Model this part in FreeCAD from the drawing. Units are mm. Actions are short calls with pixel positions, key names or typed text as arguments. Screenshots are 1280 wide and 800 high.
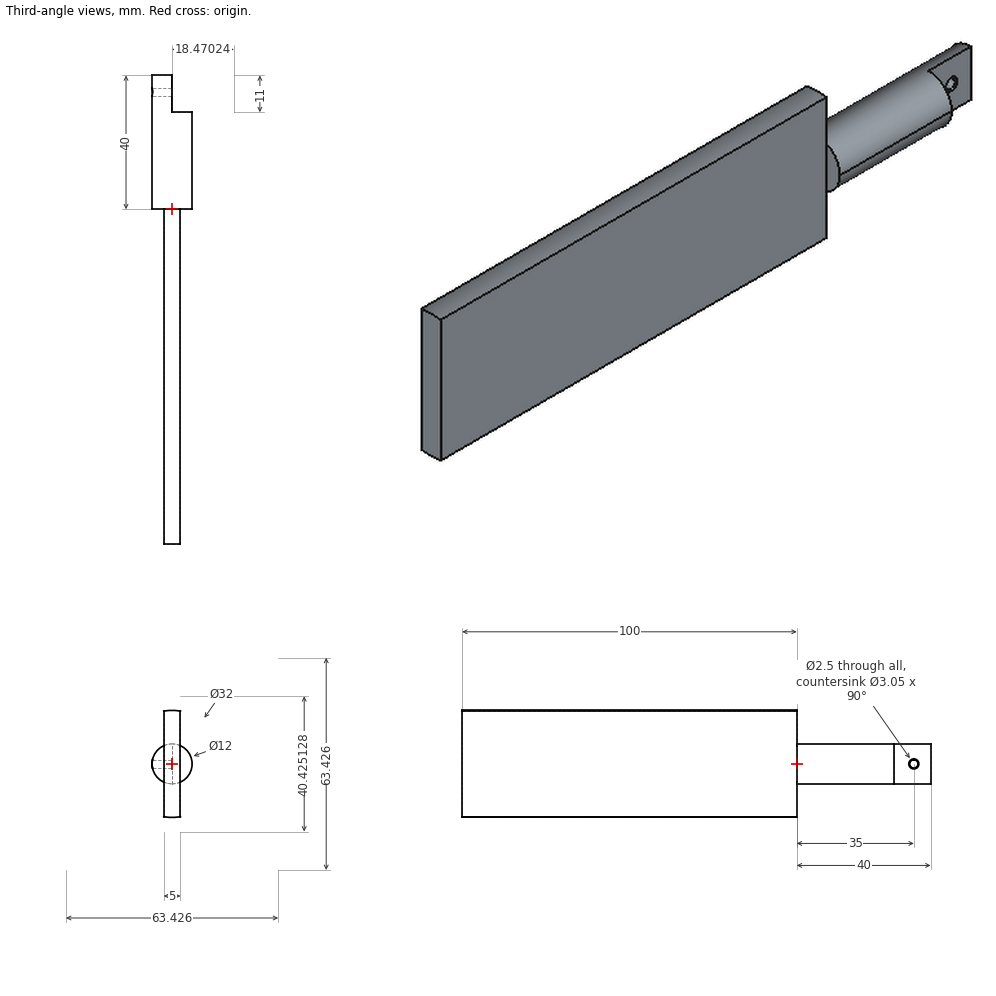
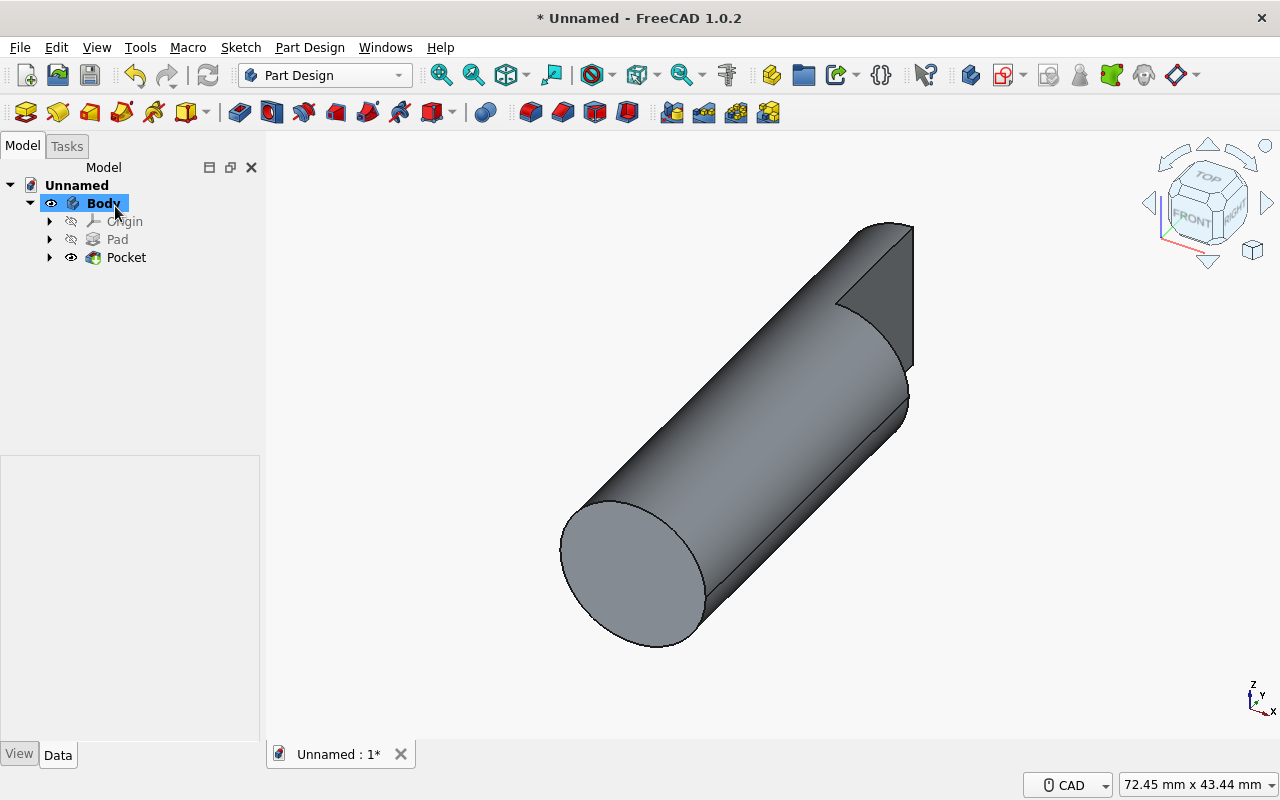
click(1004, 76)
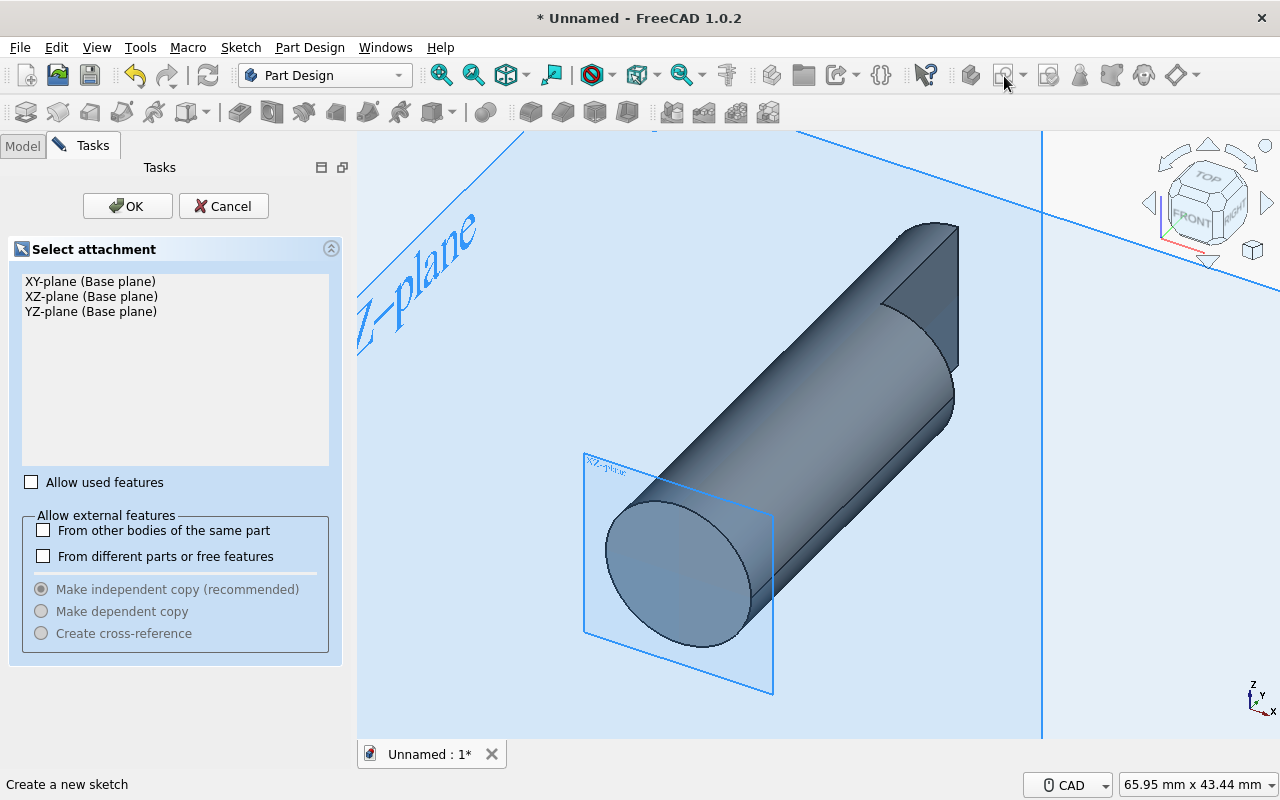
click(82, 312)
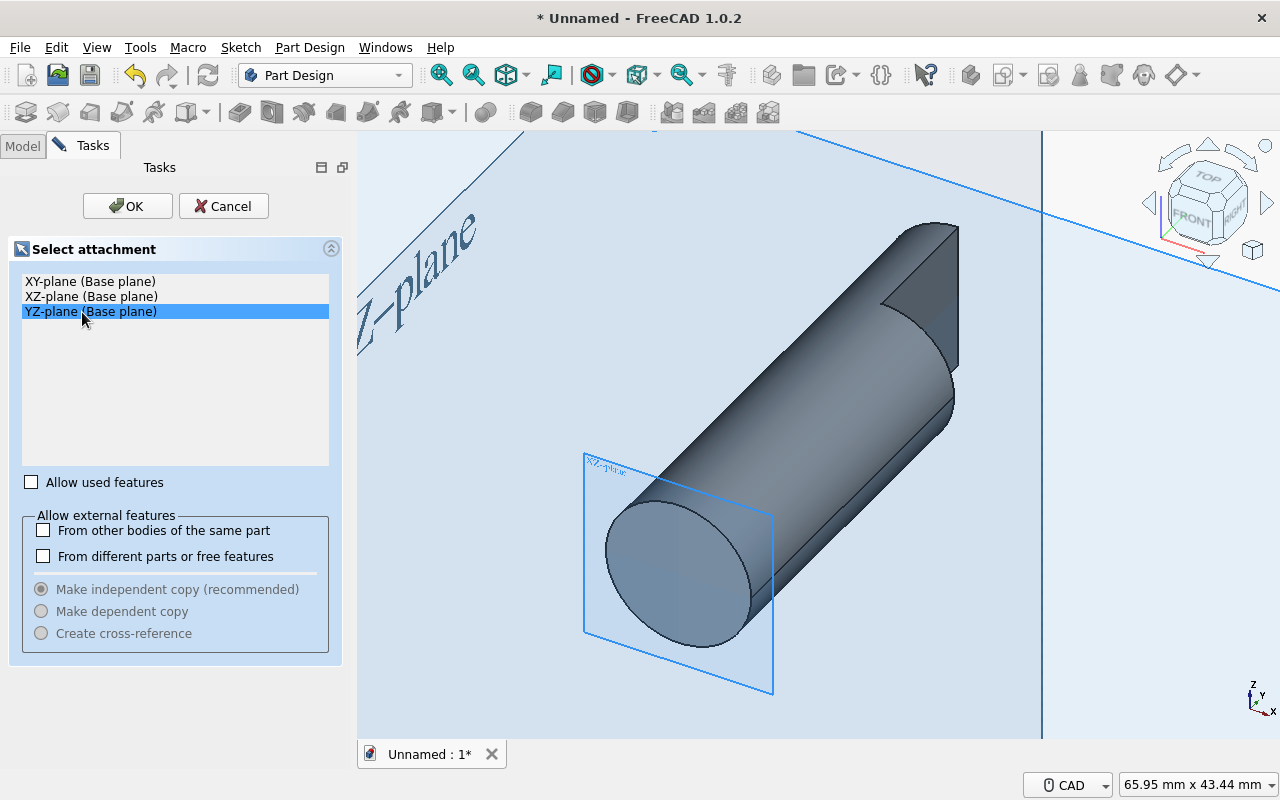
click(128, 206)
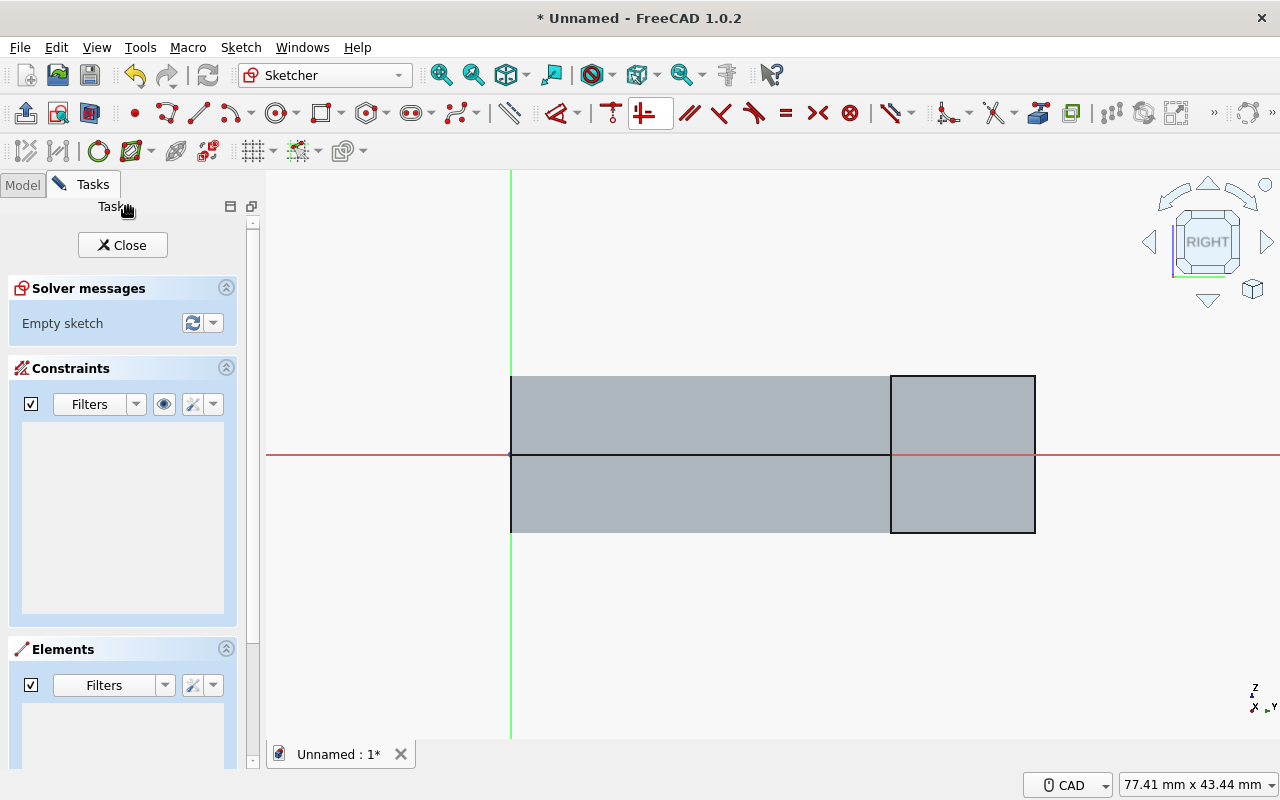
key(q)
key(s)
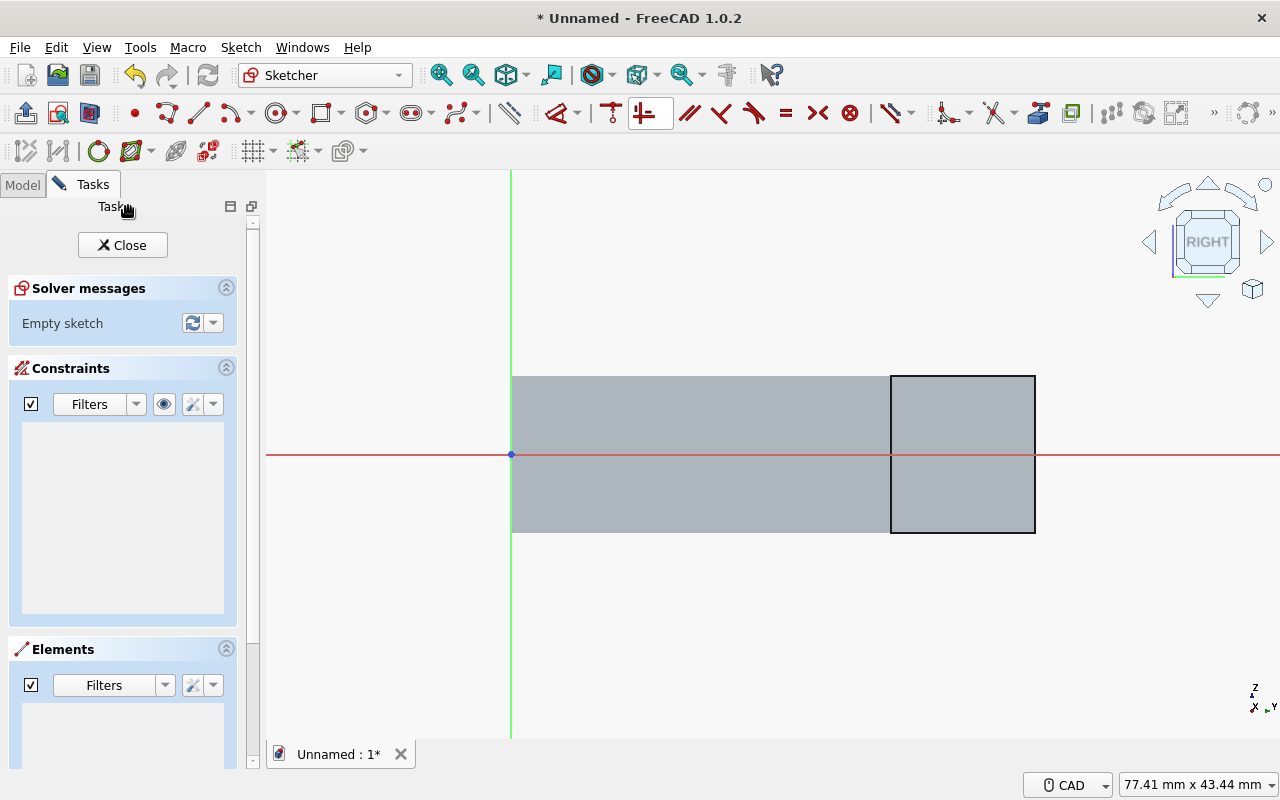
scroll(996, 455, up, 12)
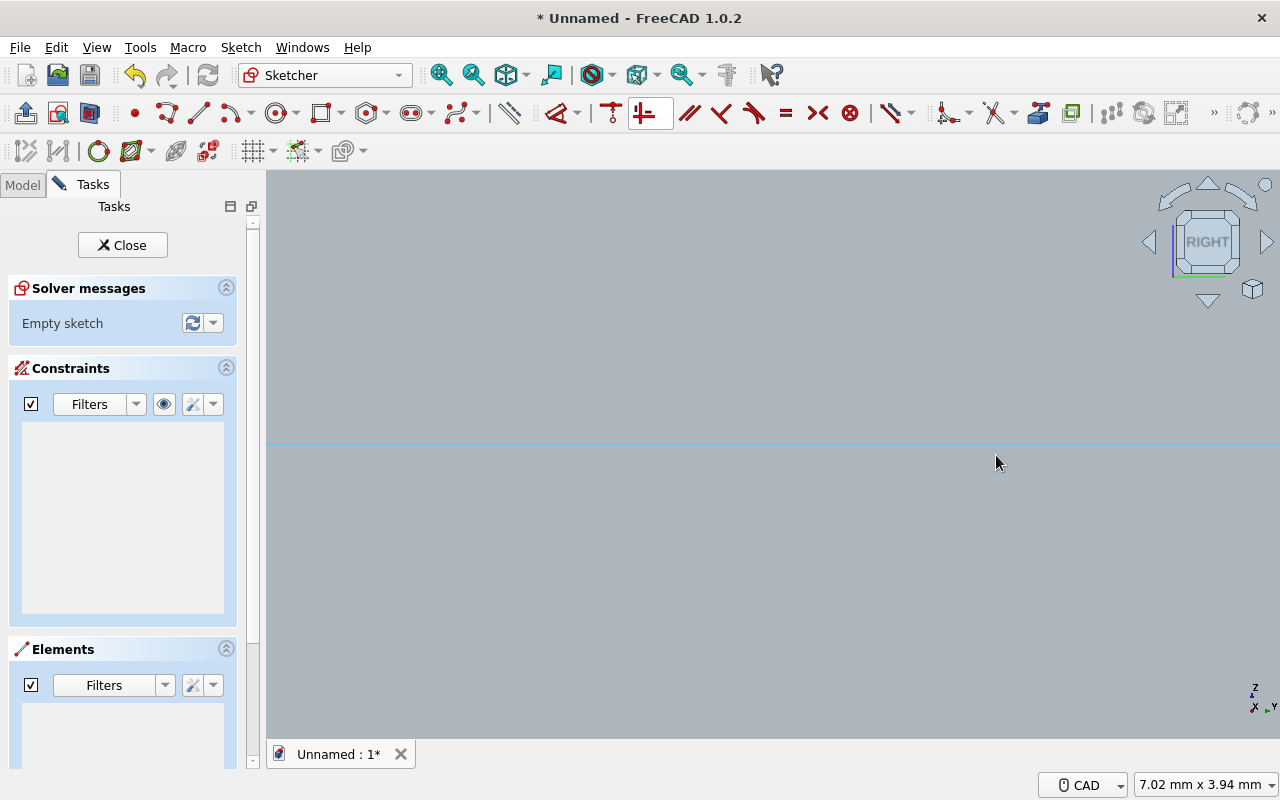
key(g)
key(c)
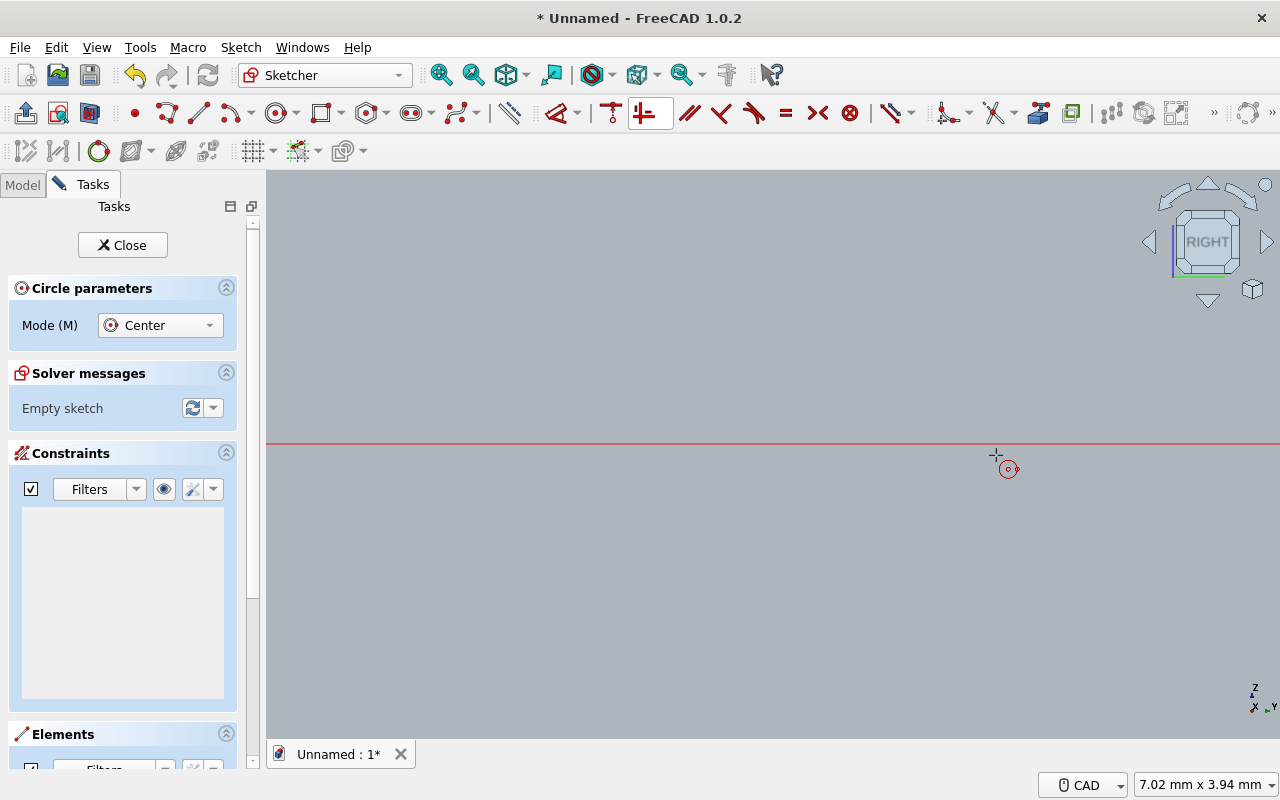
click(696, 444)
move(824, 317)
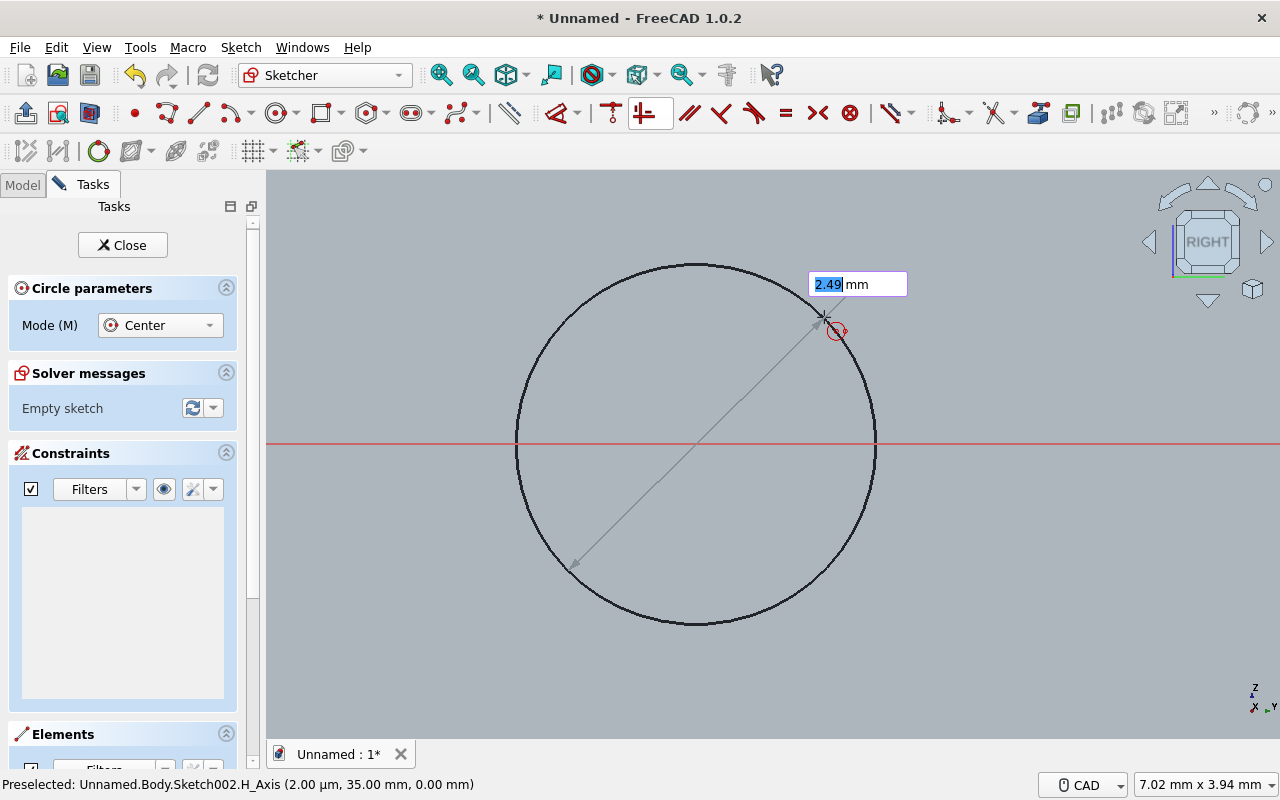
text(2.5)
key(Return)
key(Escape)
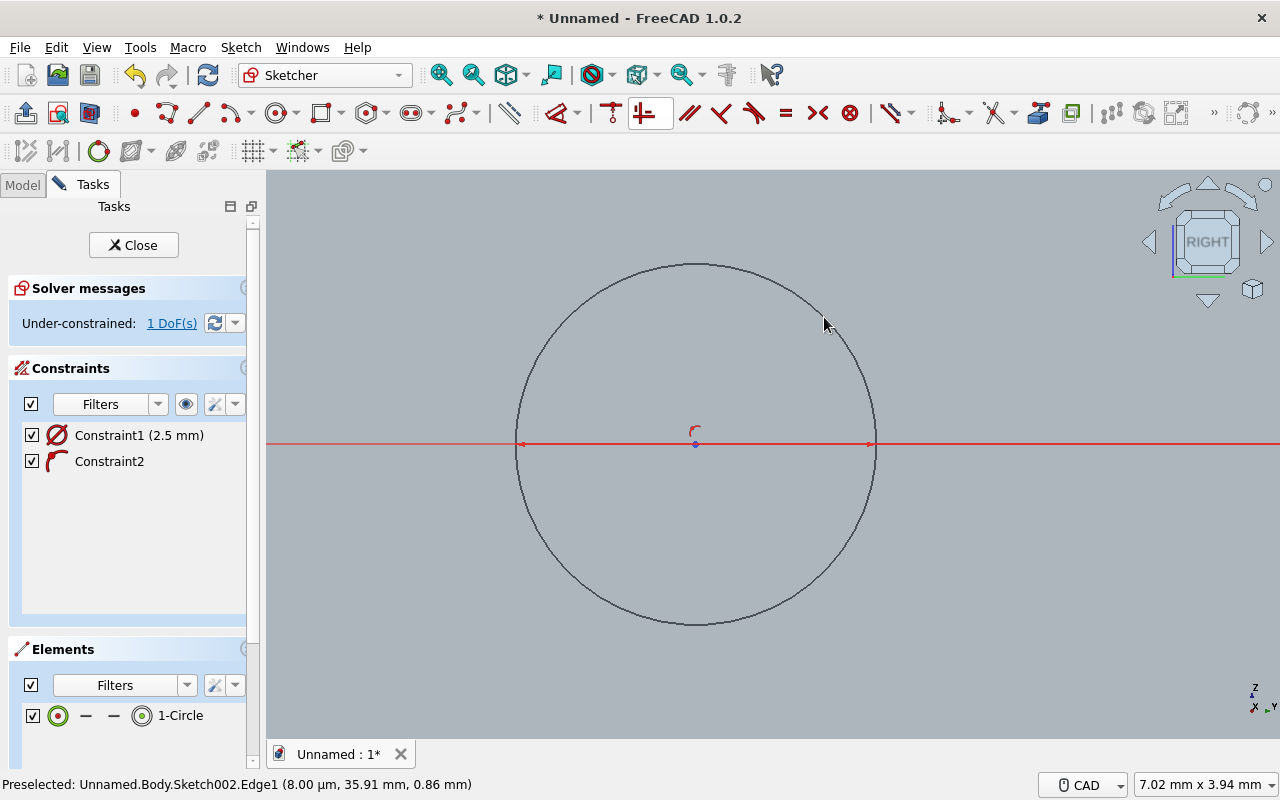
click(696, 444)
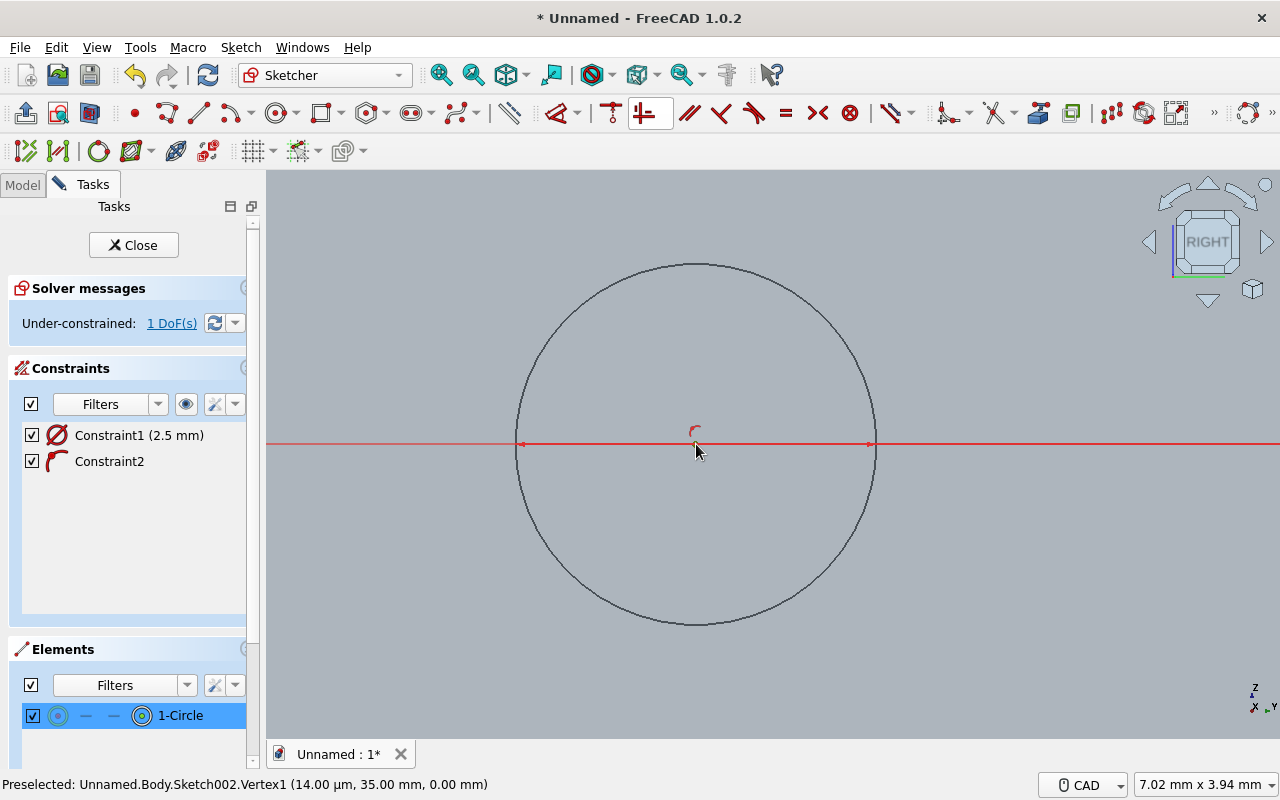
click(580, 114)